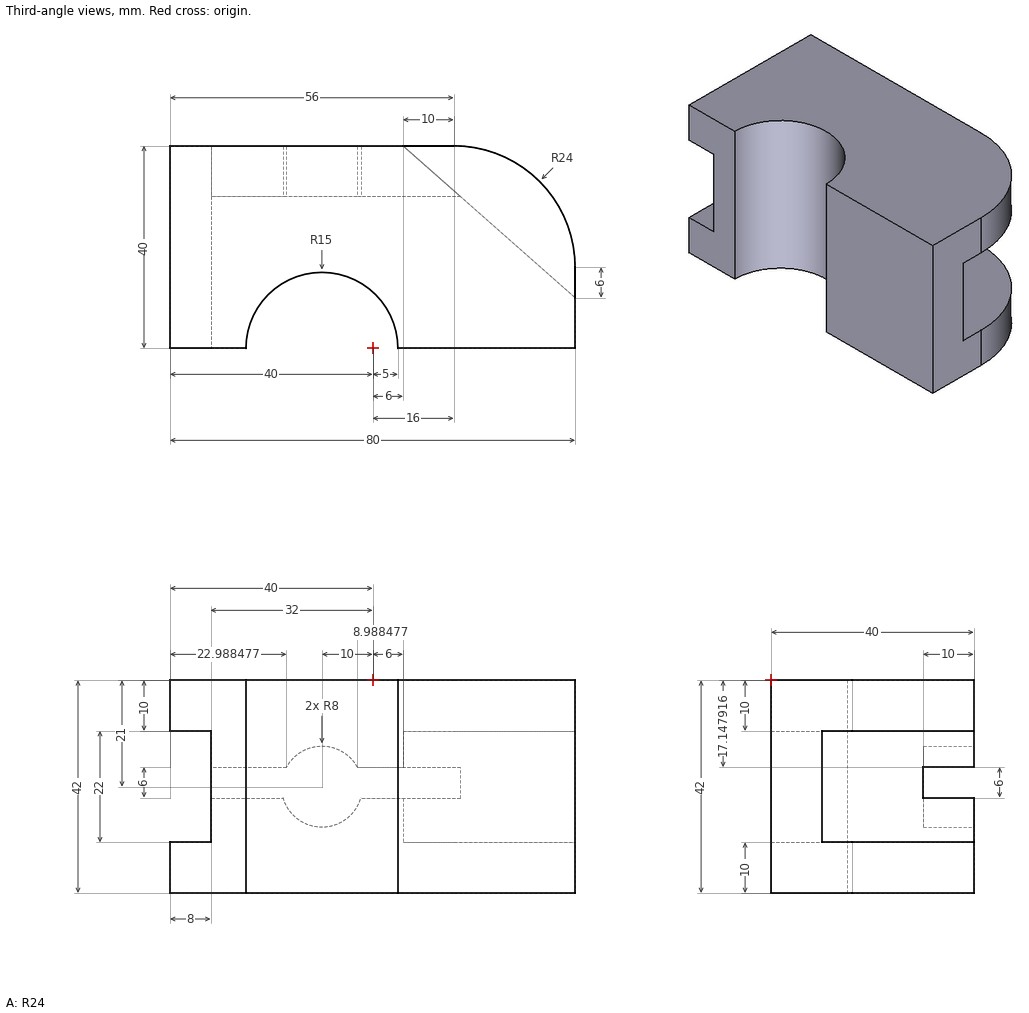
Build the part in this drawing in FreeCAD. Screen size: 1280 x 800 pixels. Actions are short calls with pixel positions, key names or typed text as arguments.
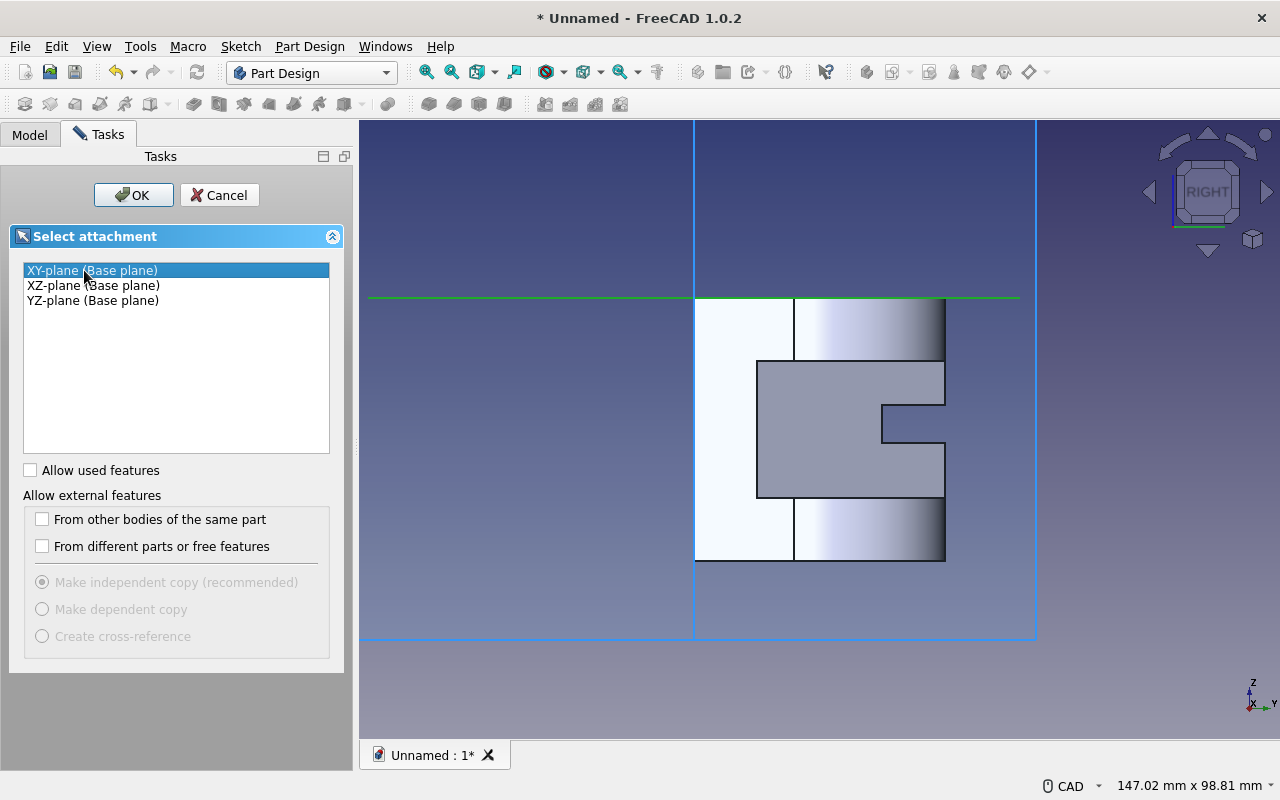
click(134, 195)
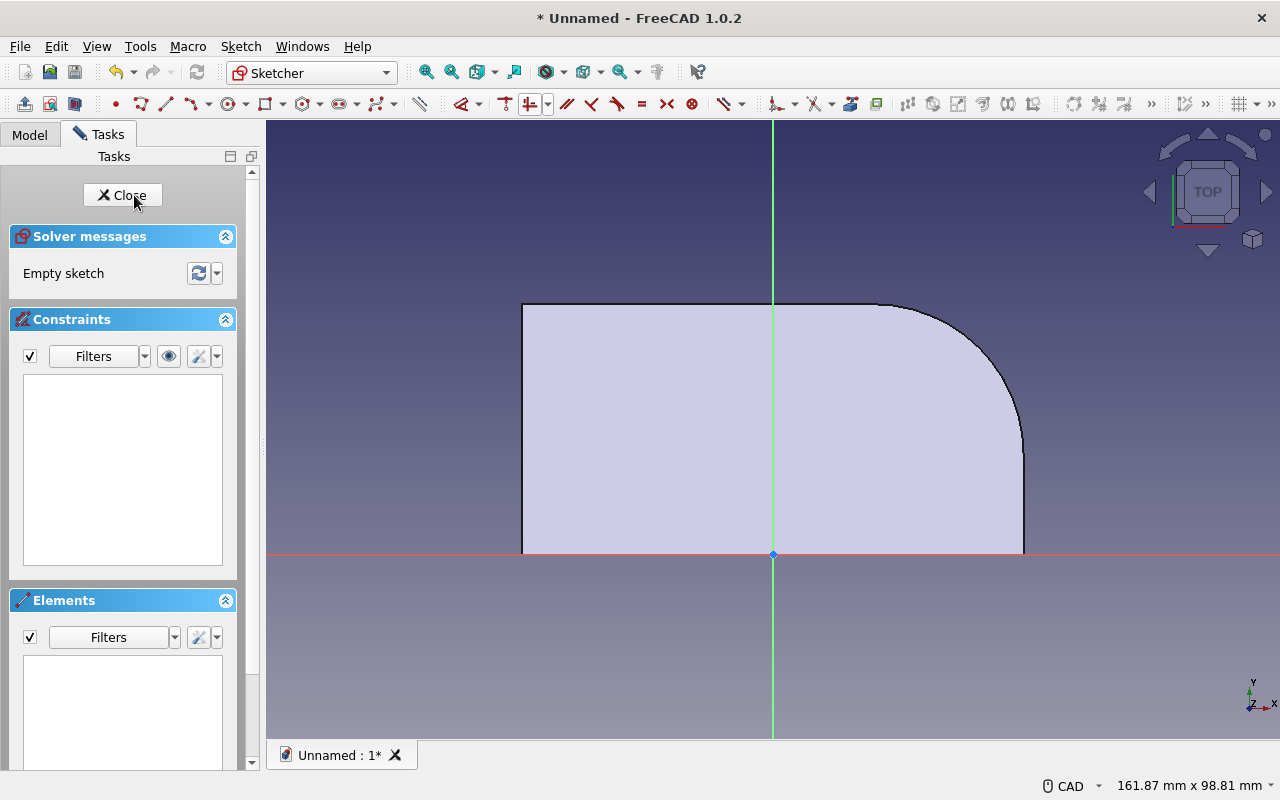
scroll(713, 542, up, 6)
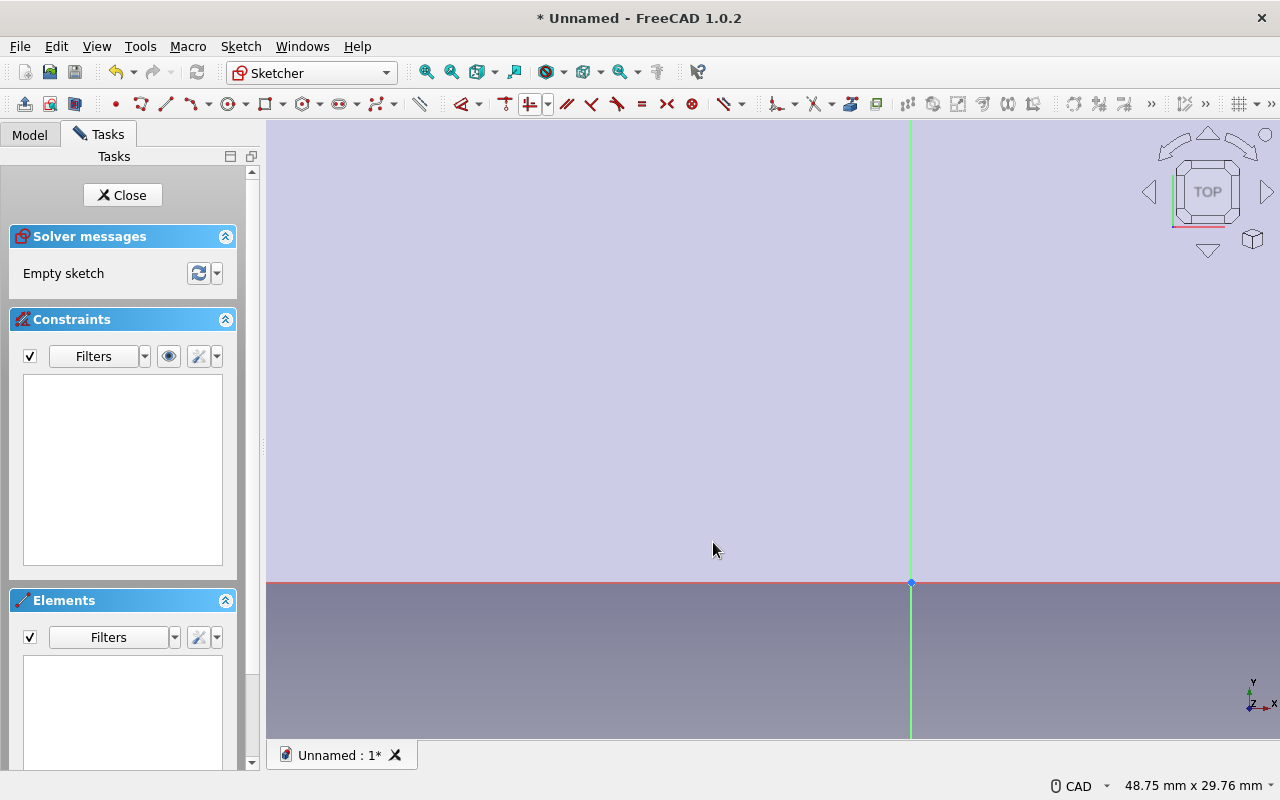
key(g)
key(l)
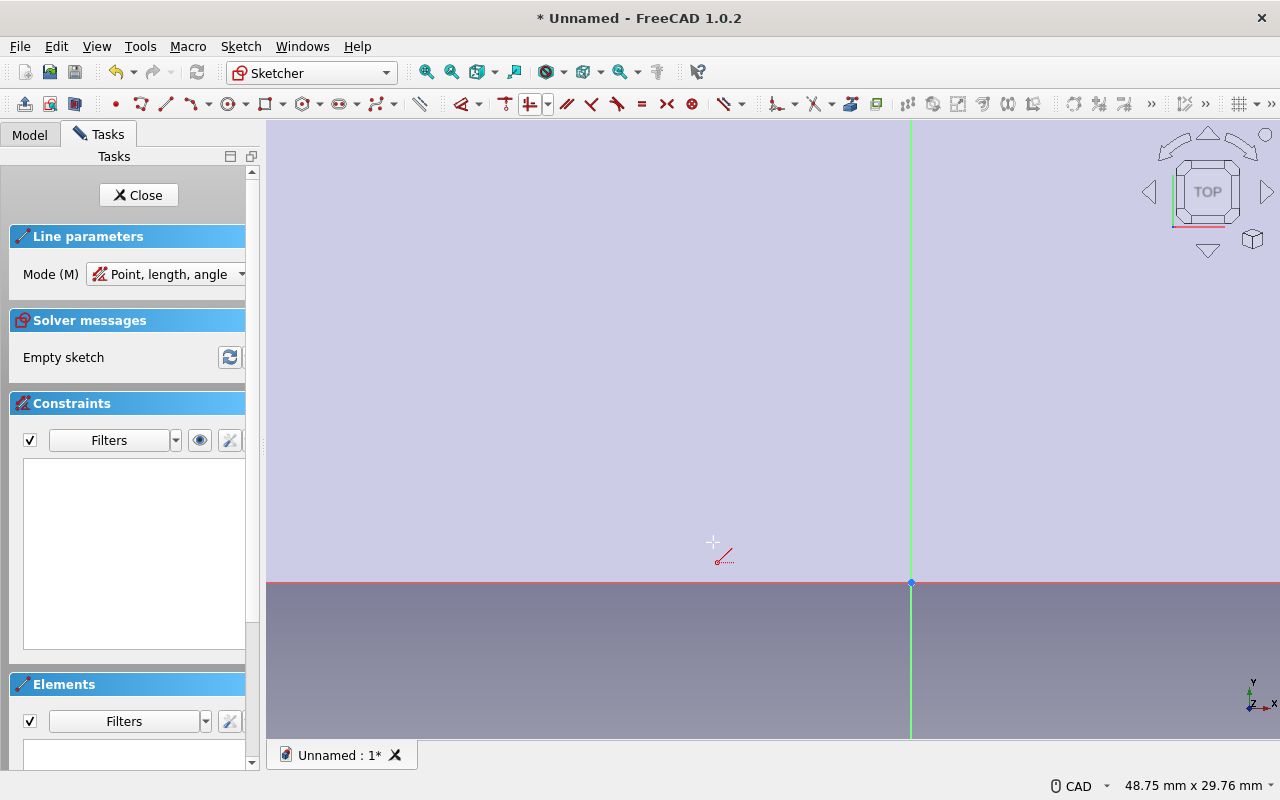
click(391, 583)
click(1015, 574)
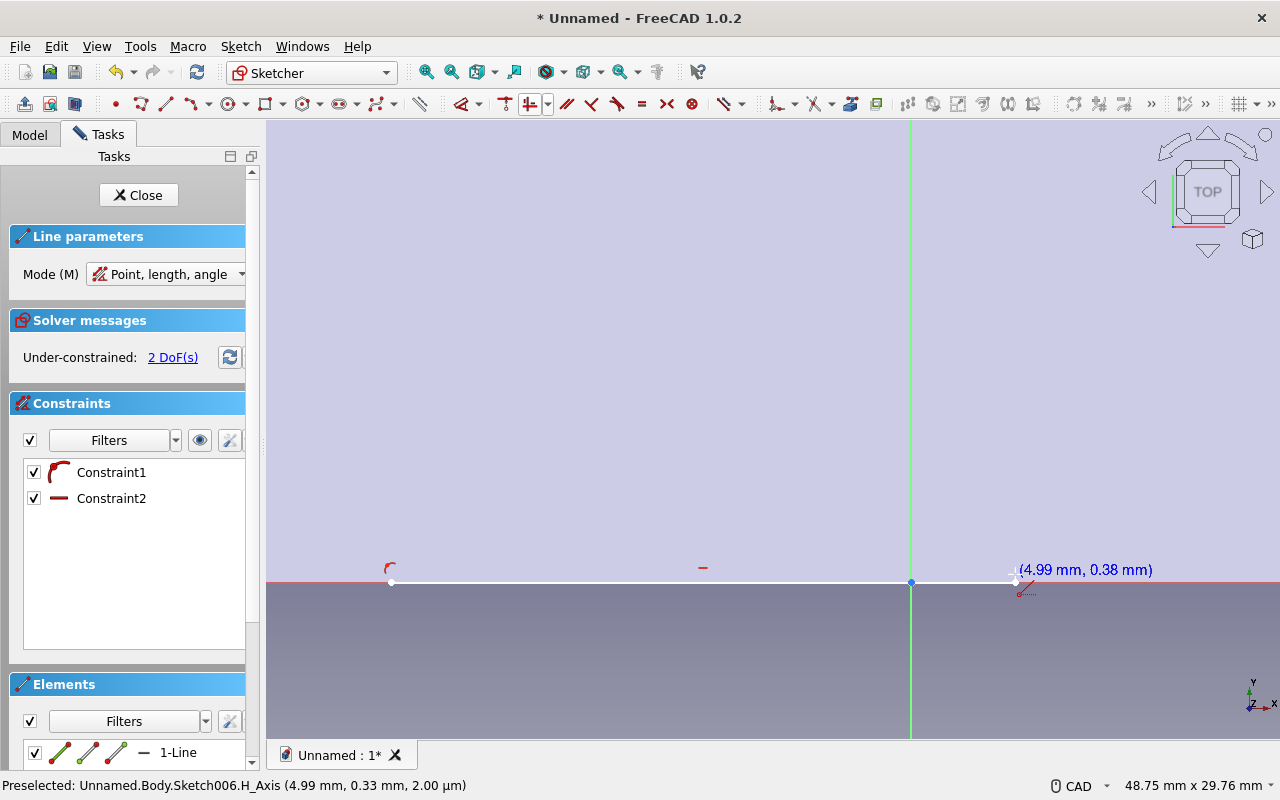
key(g)
key(3)
key(a)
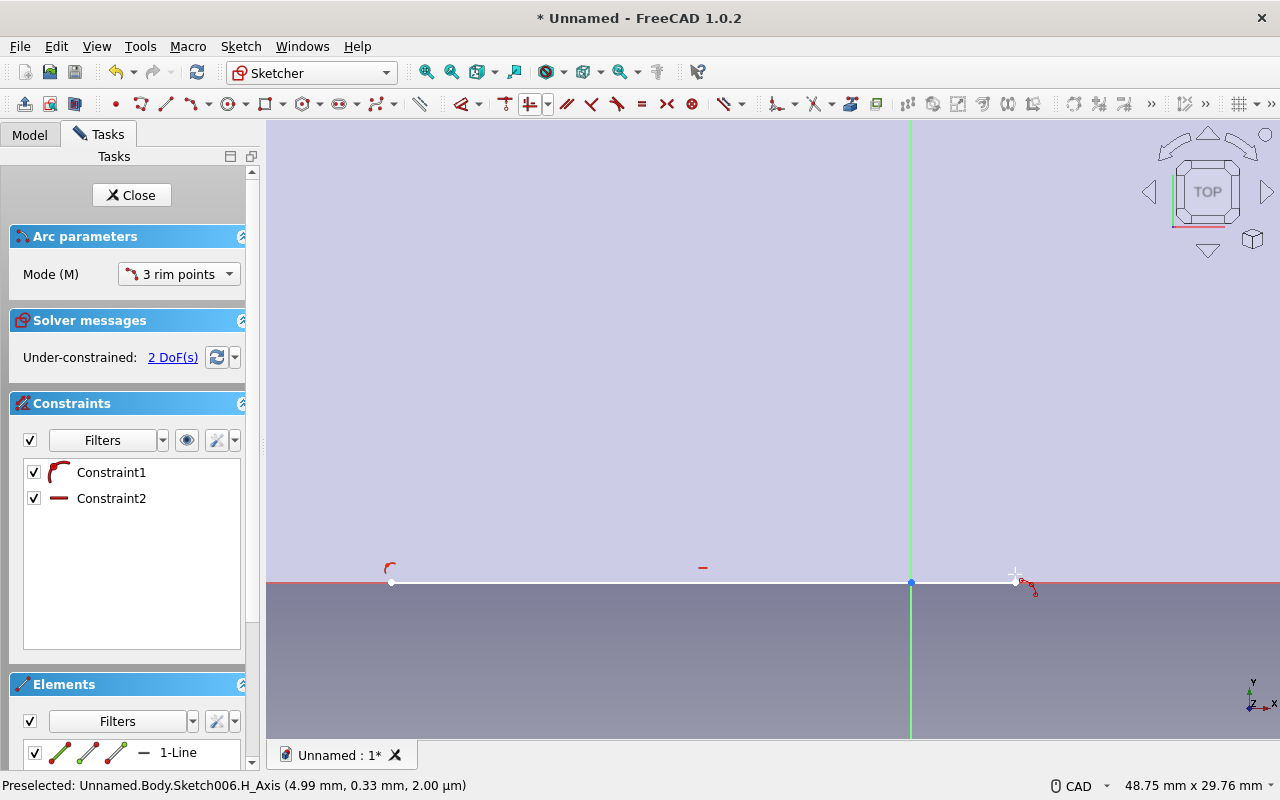
click(1015, 583)
click(391, 583)
click(703, 271)
key(Escape)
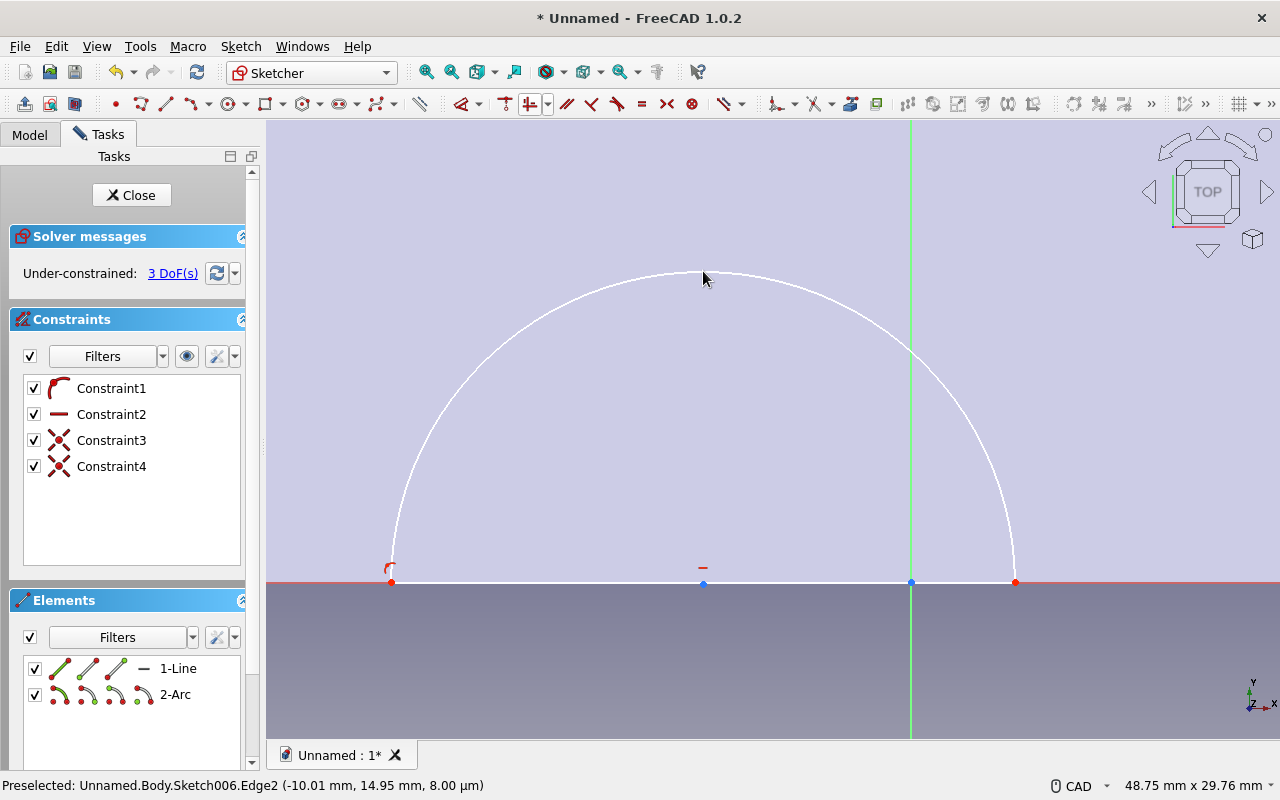
click(703, 584)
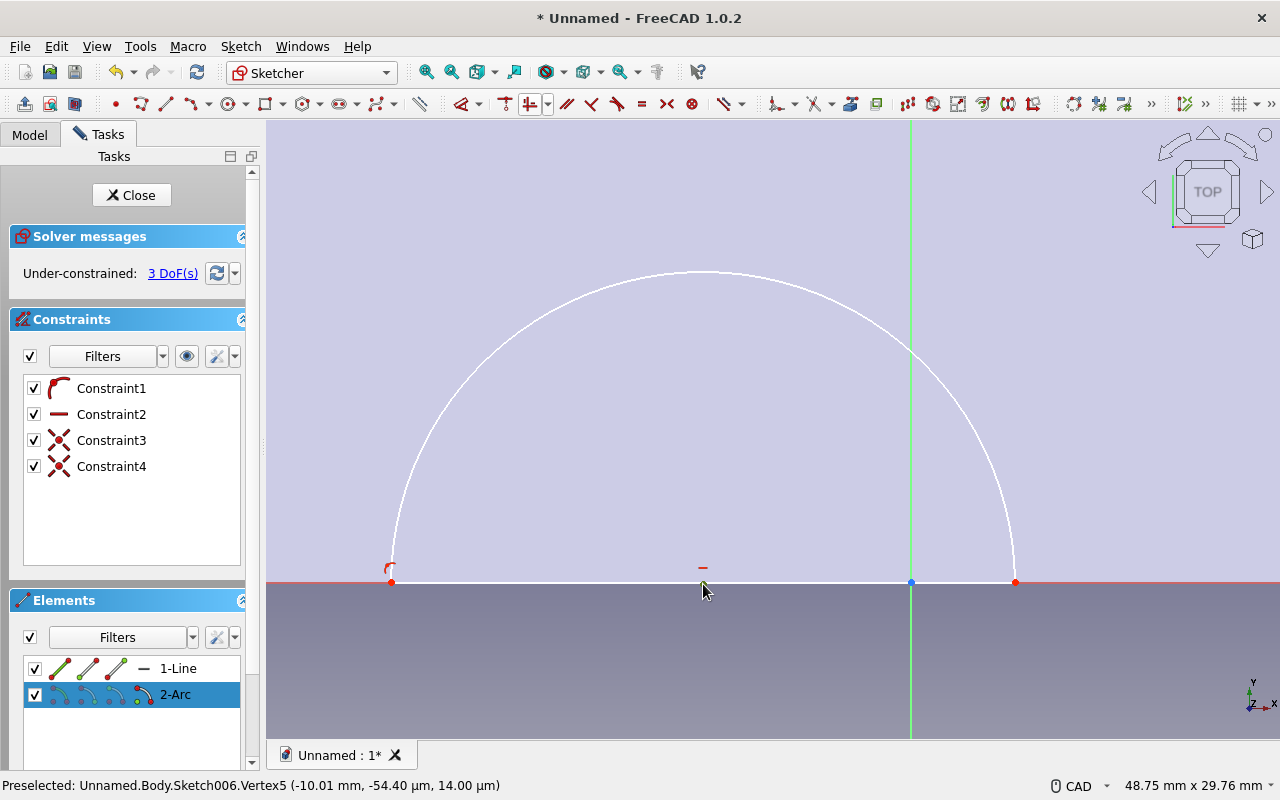
click(353, 583)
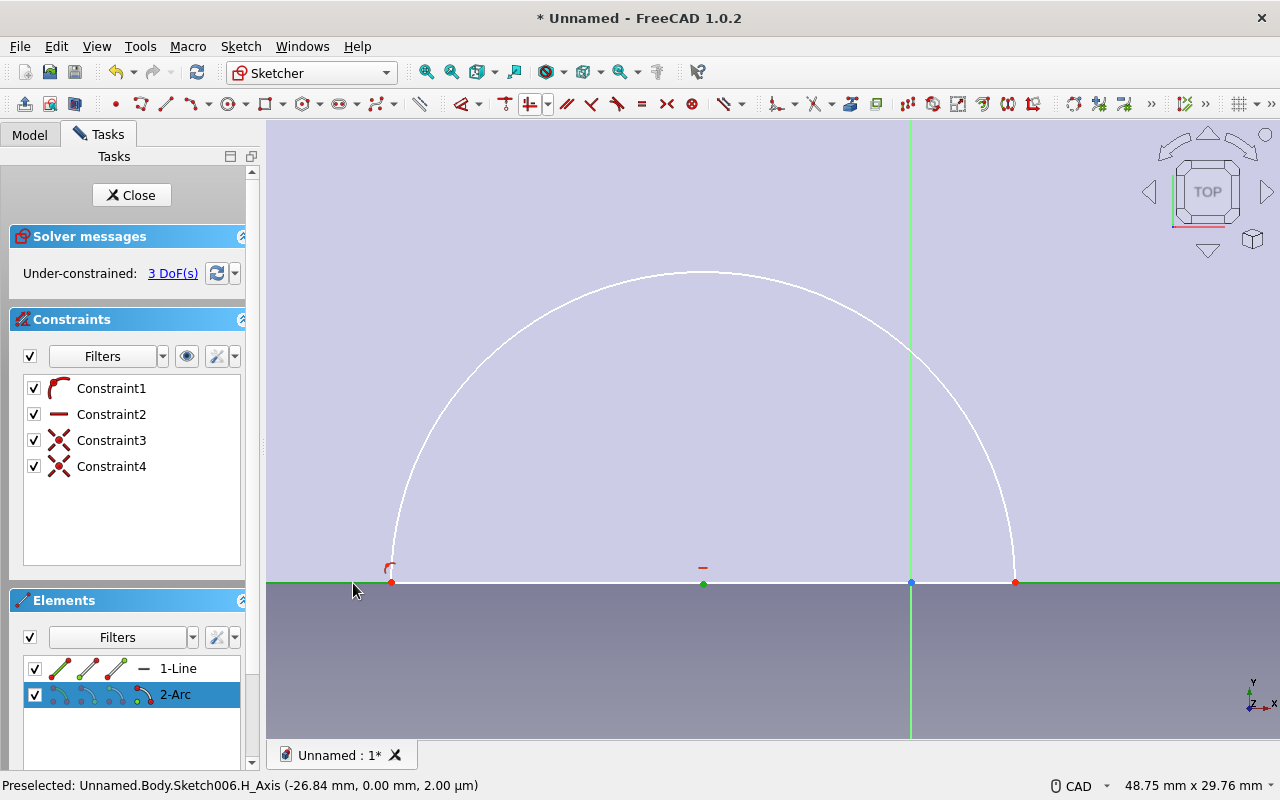
click(505, 104)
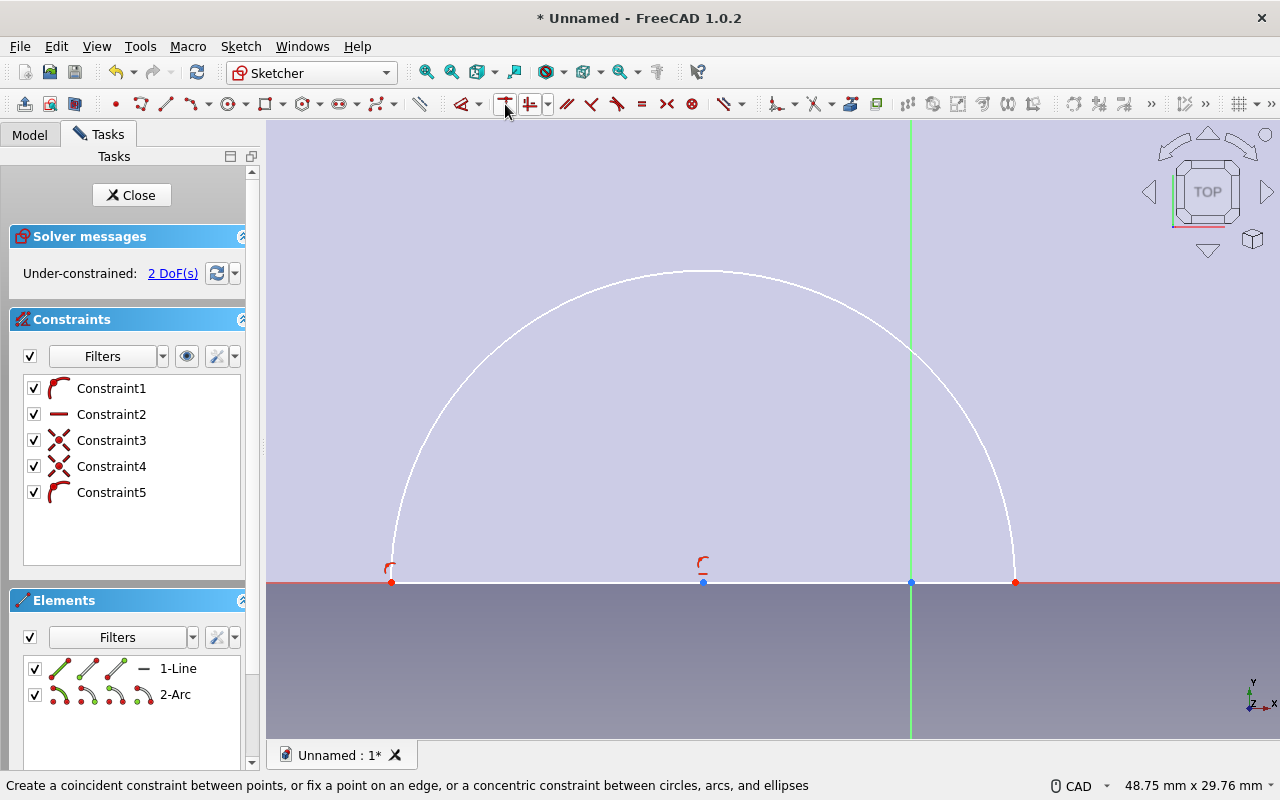
click(460, 104)